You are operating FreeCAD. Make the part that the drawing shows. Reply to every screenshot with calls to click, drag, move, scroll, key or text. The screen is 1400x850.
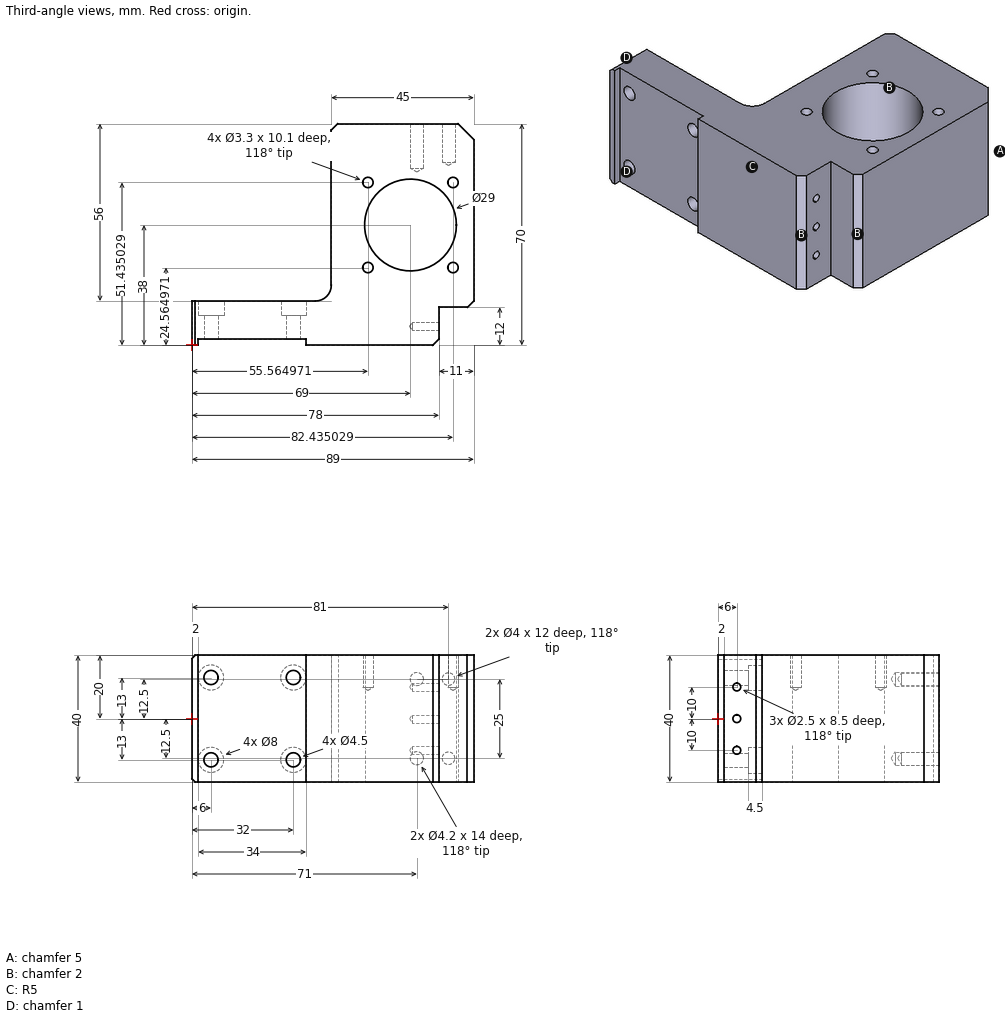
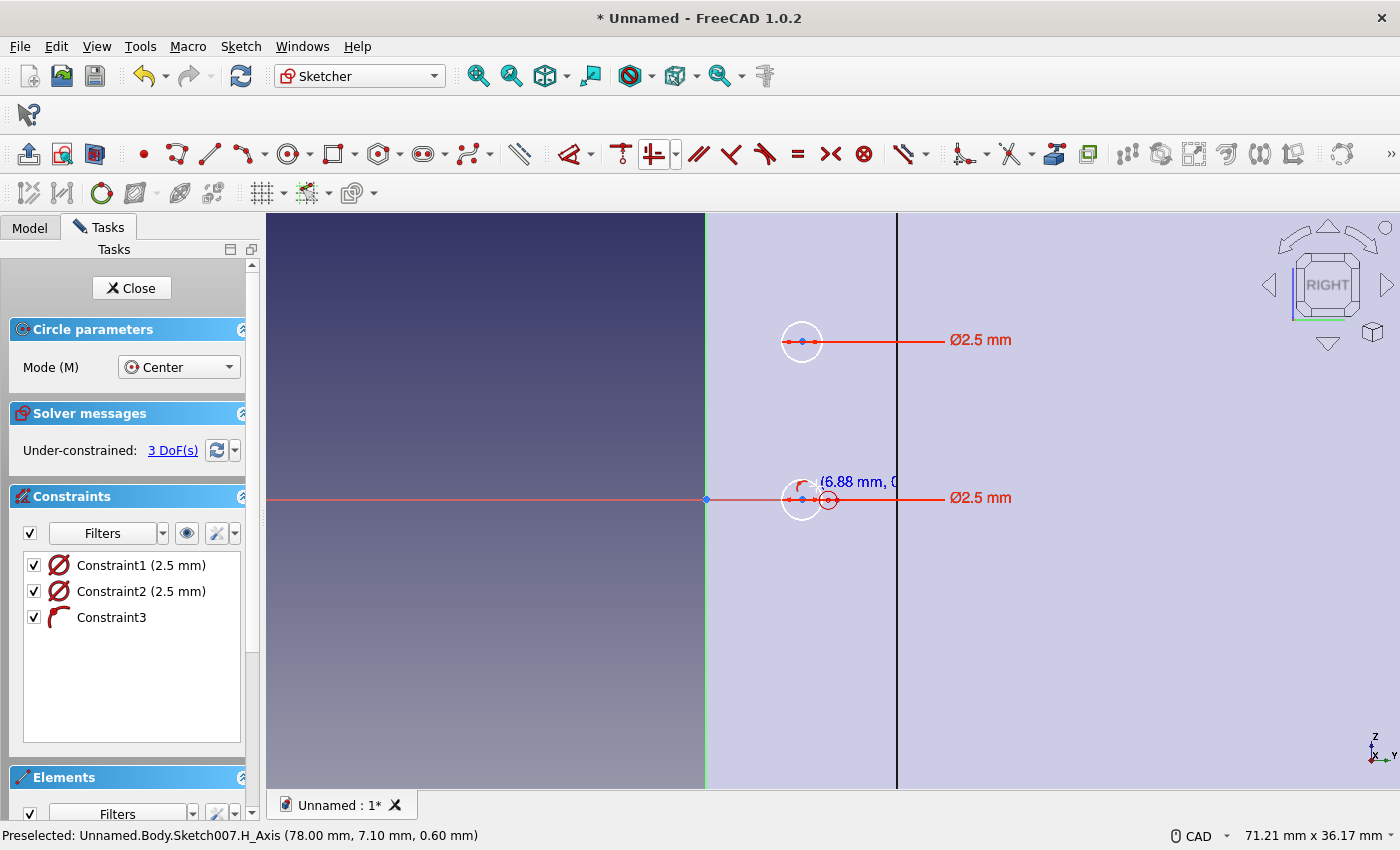
click(802, 659)
move(816, 645)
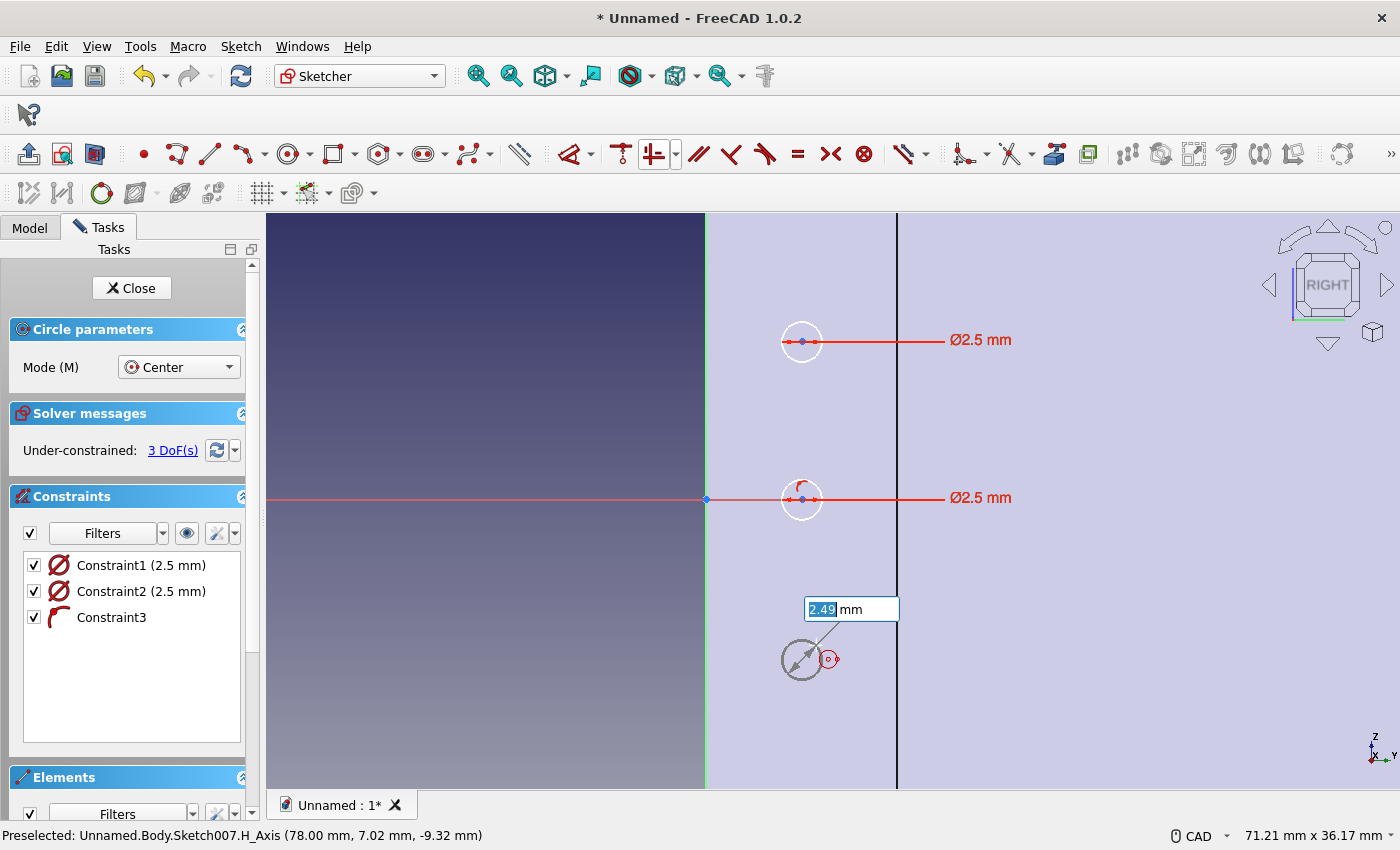
text(2.5)
key(Return)
key(Escape)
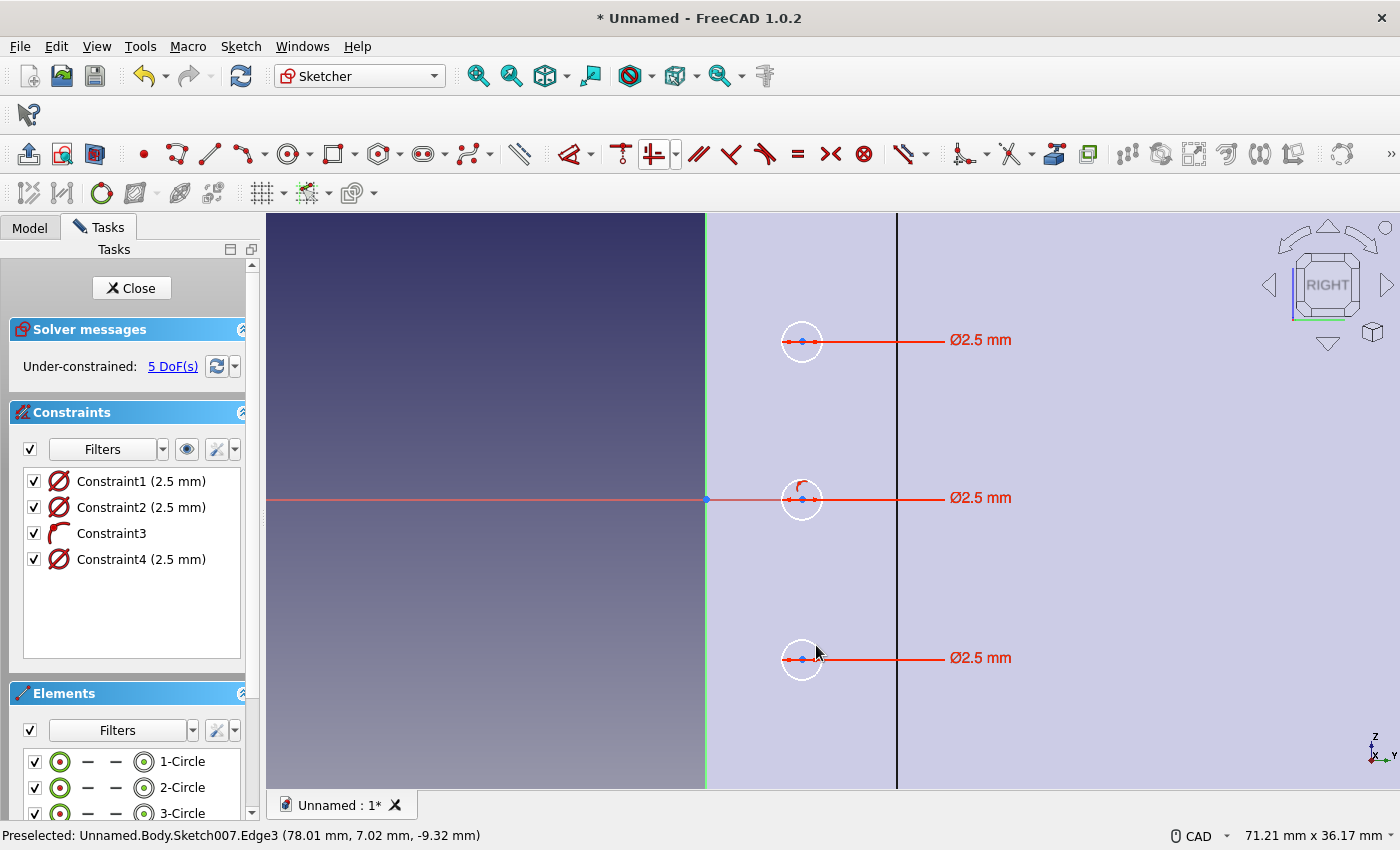
click(802, 342)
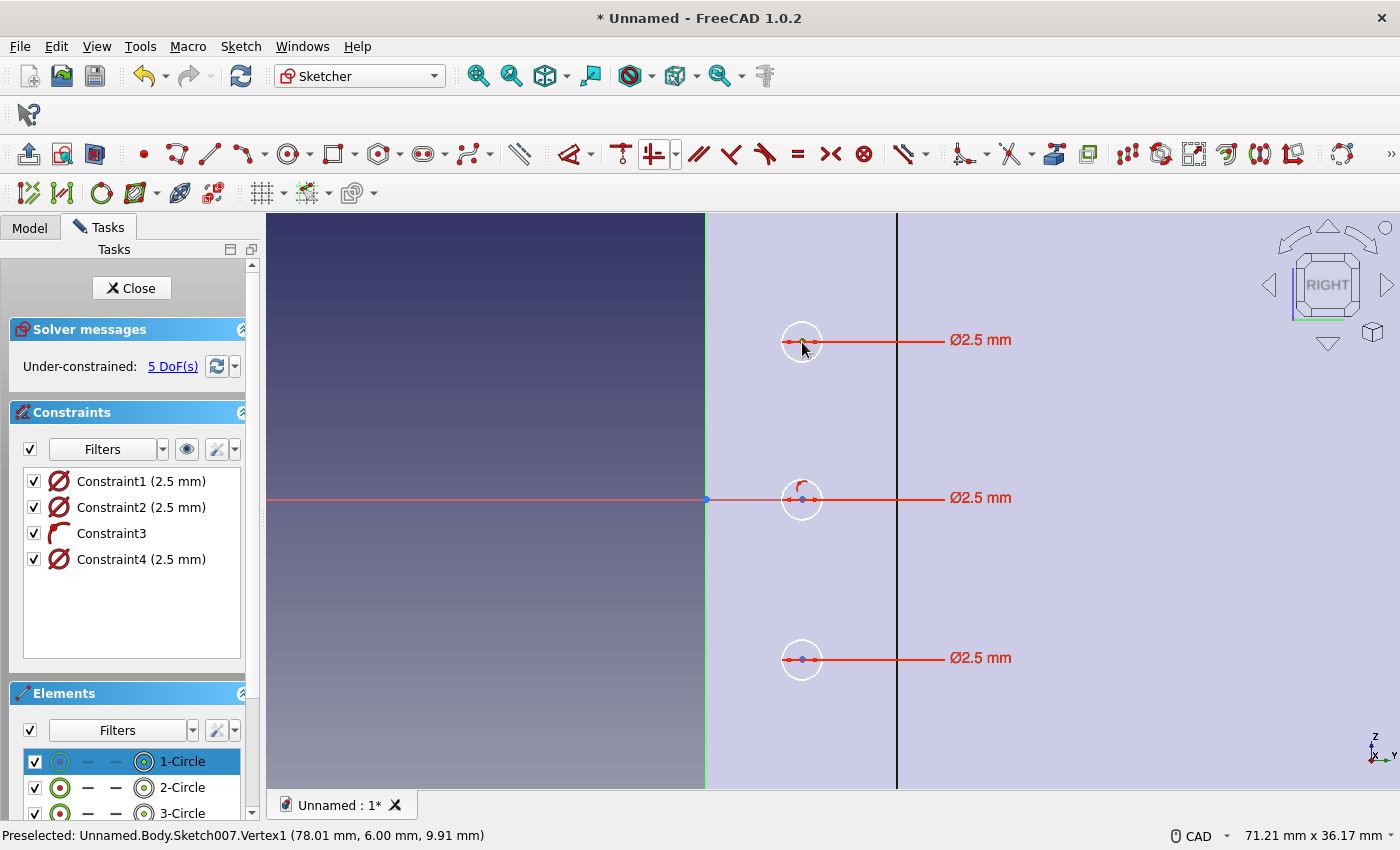
click(802, 500)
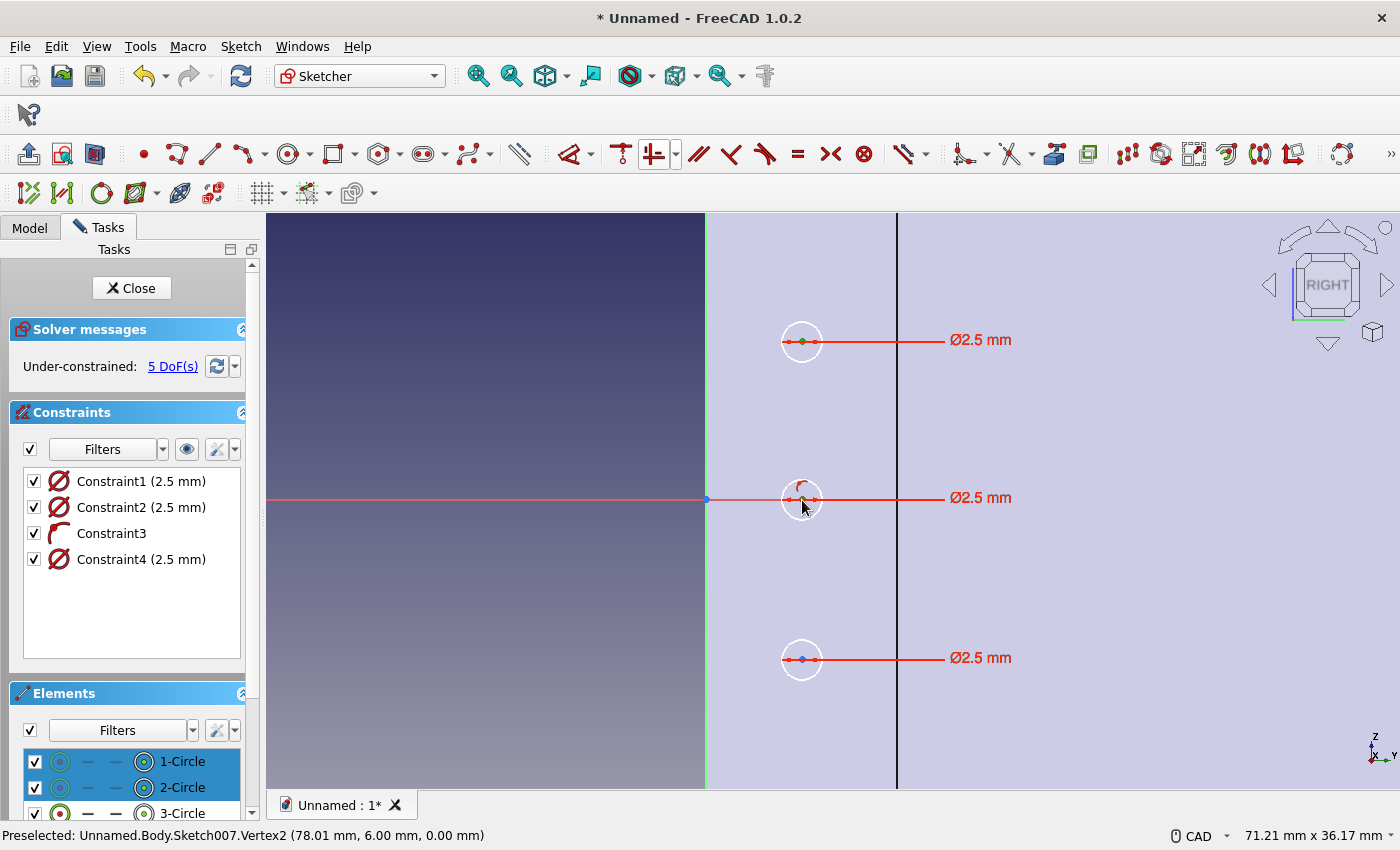
key(v)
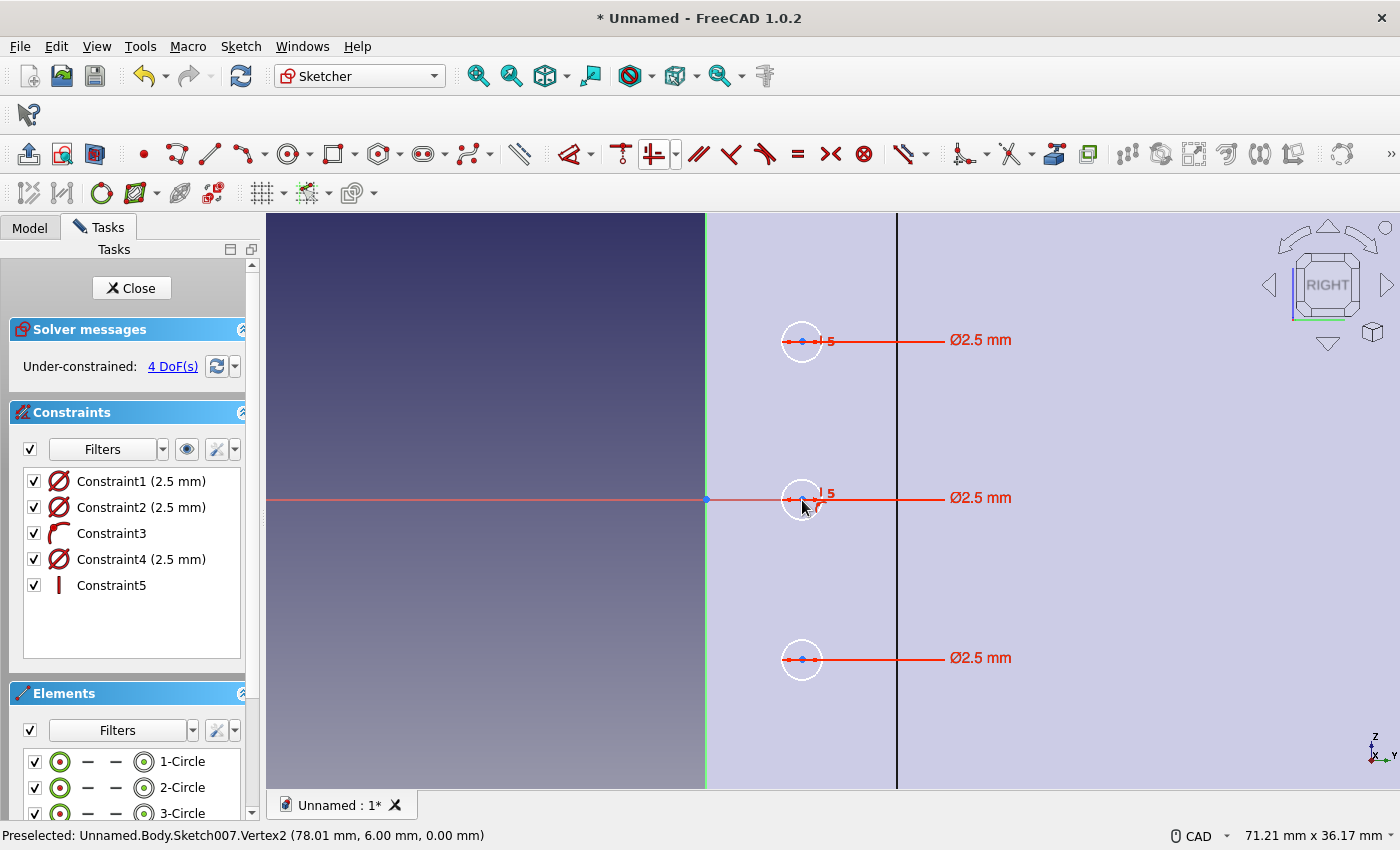
click(802, 500)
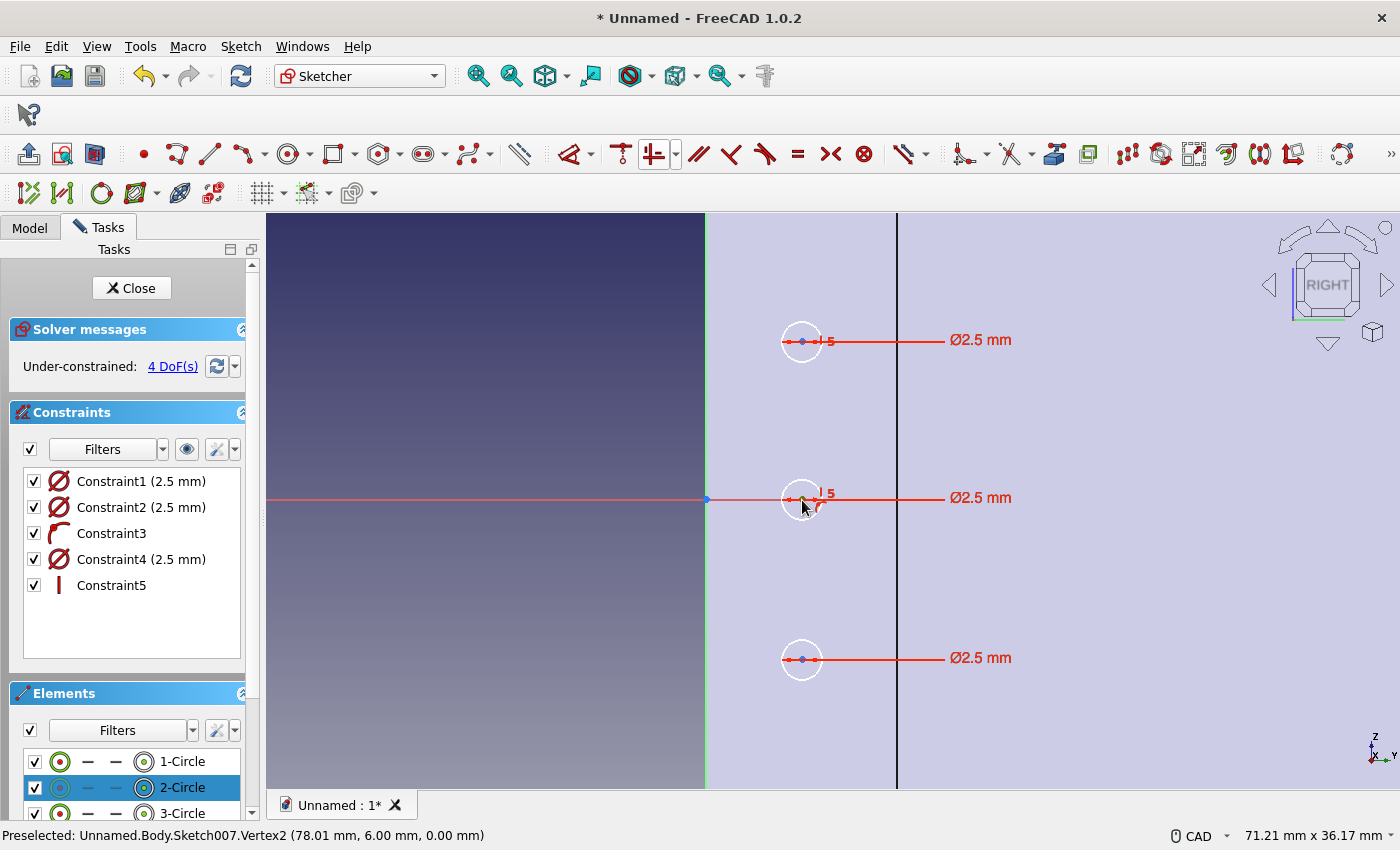
click(802, 660)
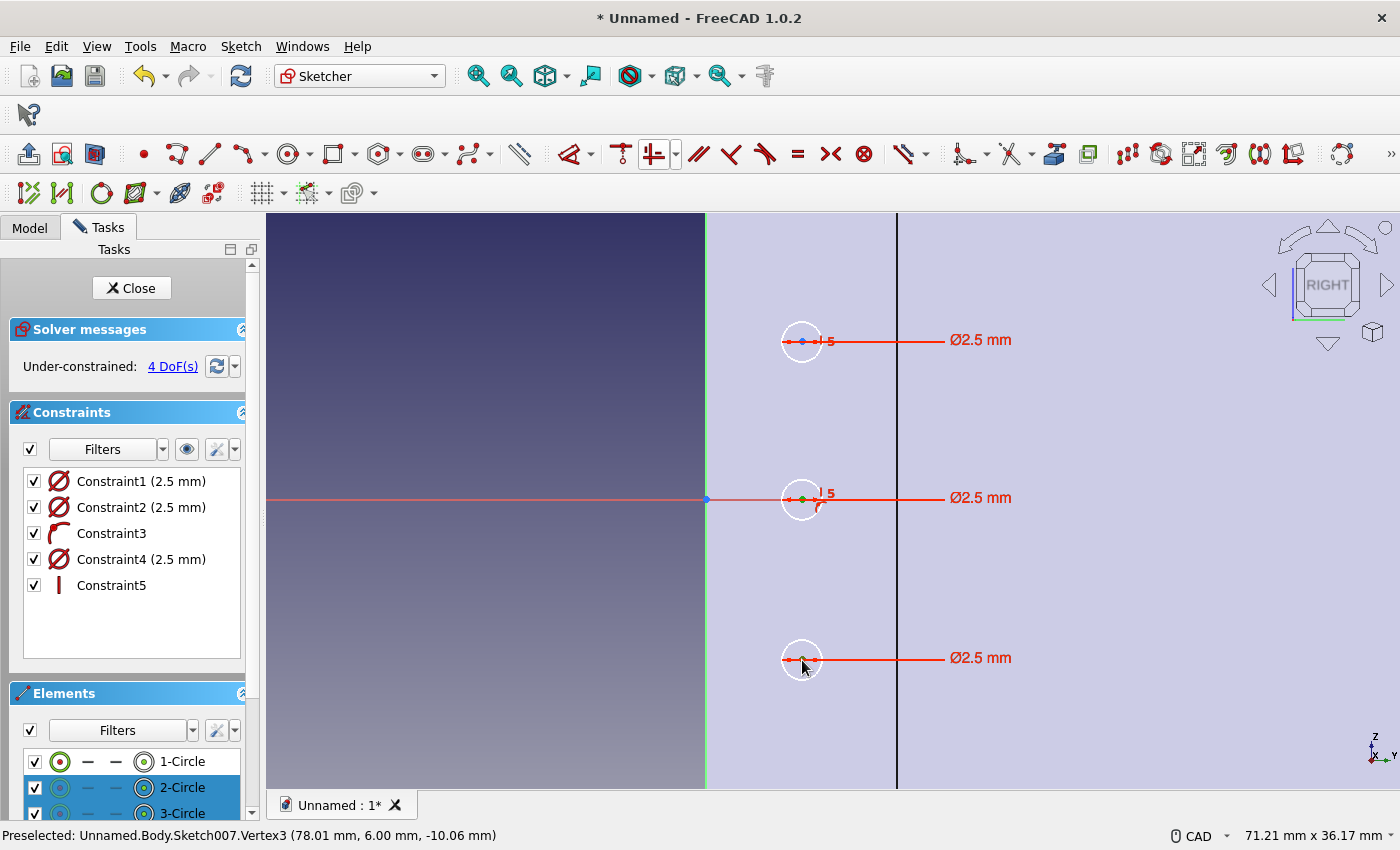
click(676, 154)